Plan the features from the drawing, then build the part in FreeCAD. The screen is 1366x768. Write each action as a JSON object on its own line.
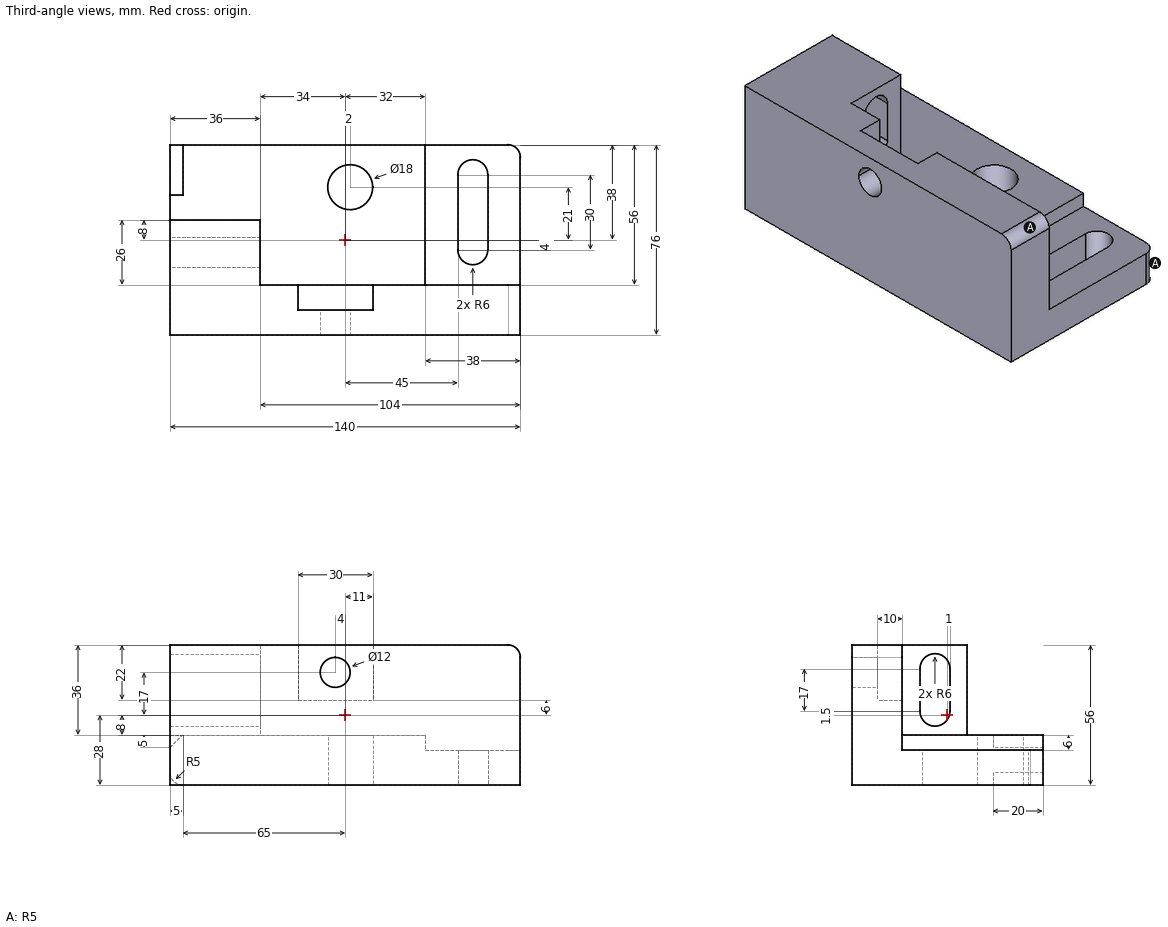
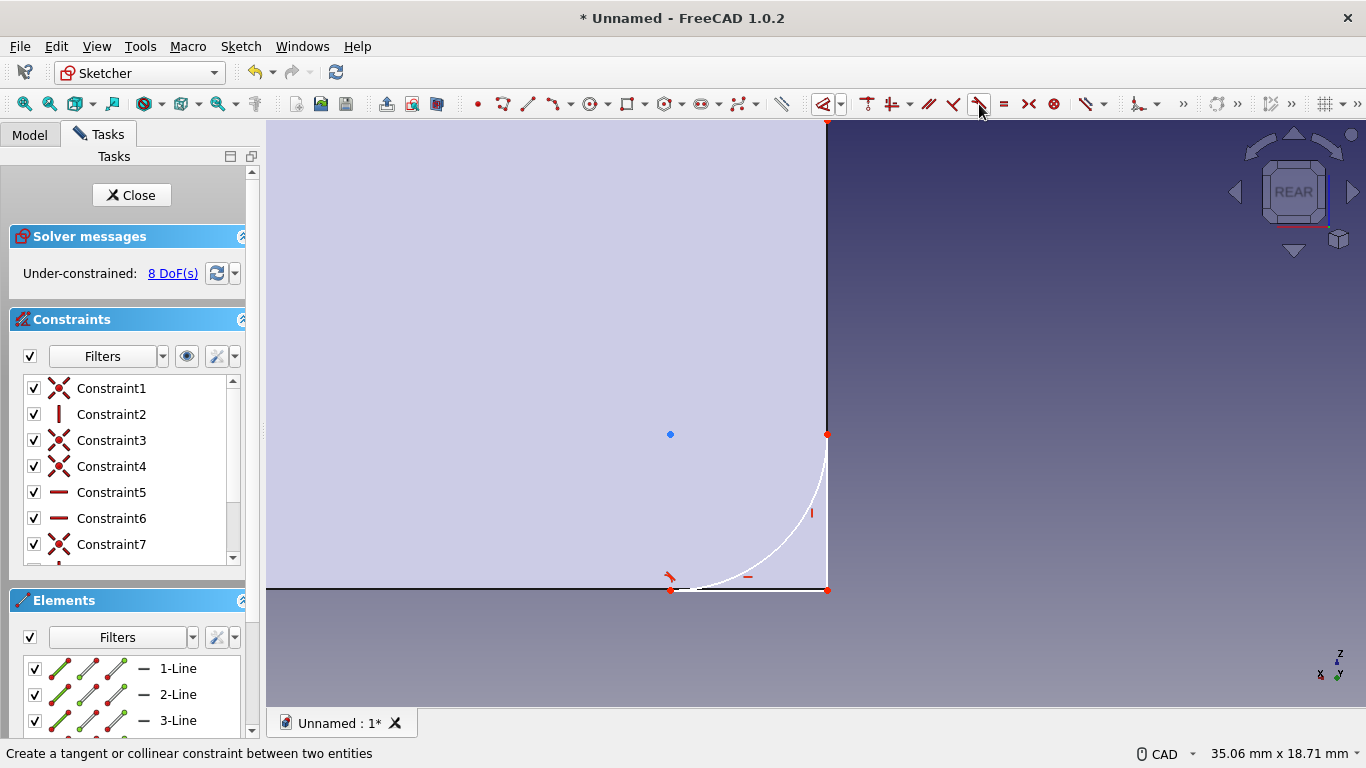
{"action": "left_click", "coordinate": [827, 544]}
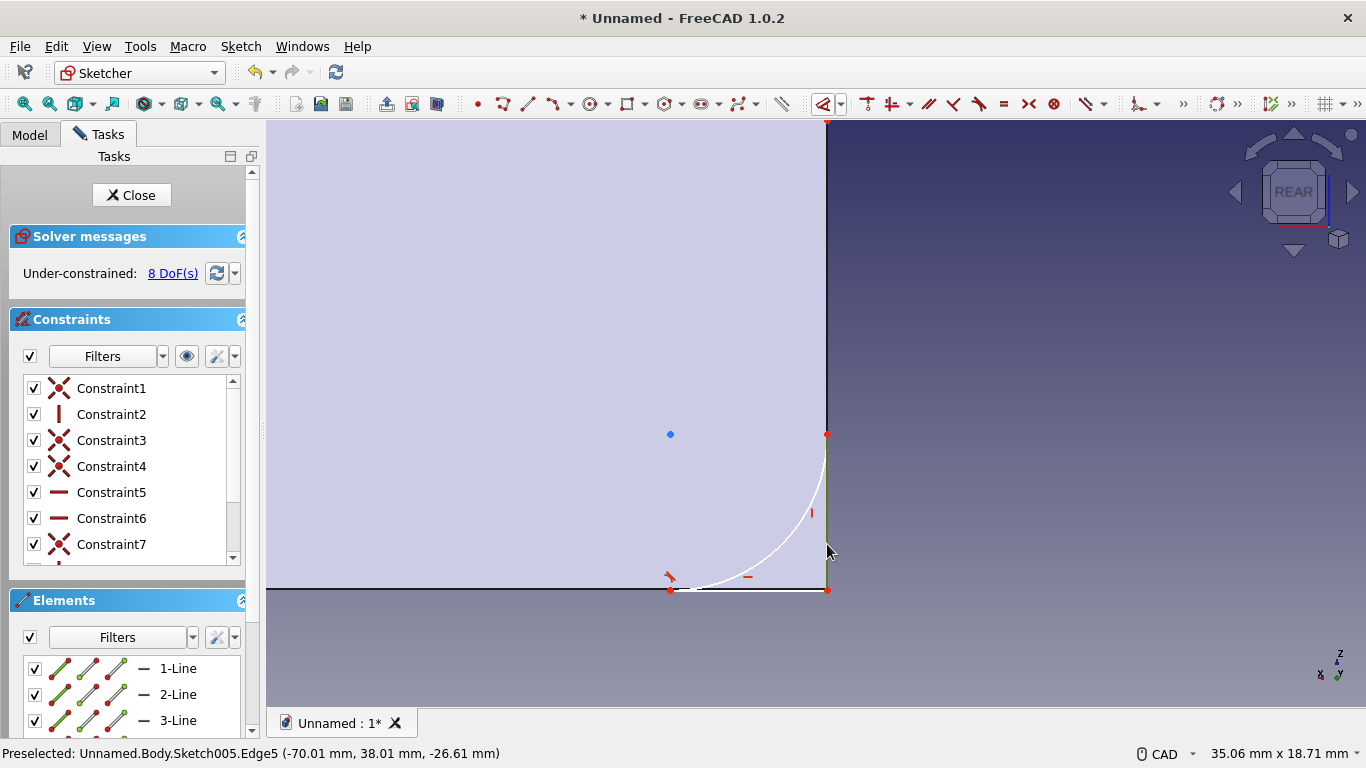
{"action": "left_click", "coordinate": [742, 574]}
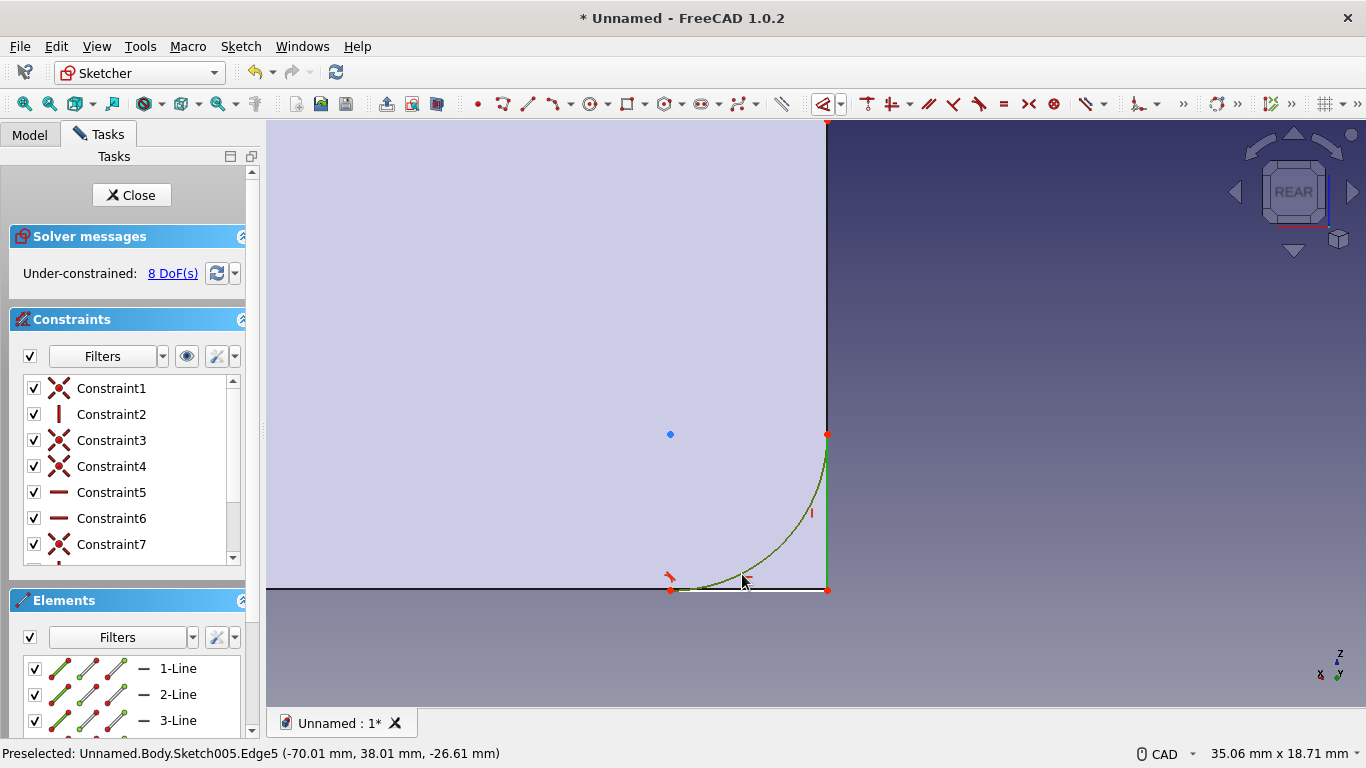
{"action": "left_click", "coordinate": [979, 104]}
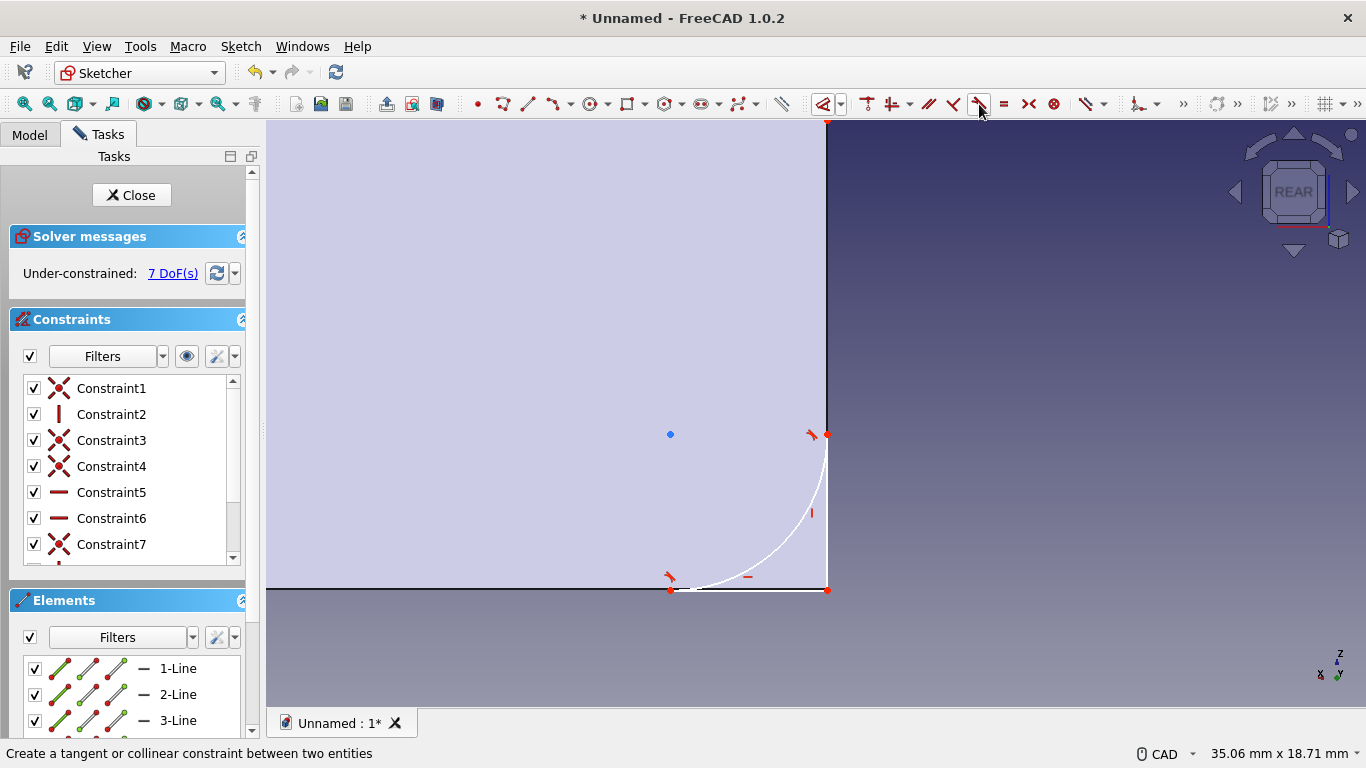
{"action": "left_click", "coordinate": [742, 574]}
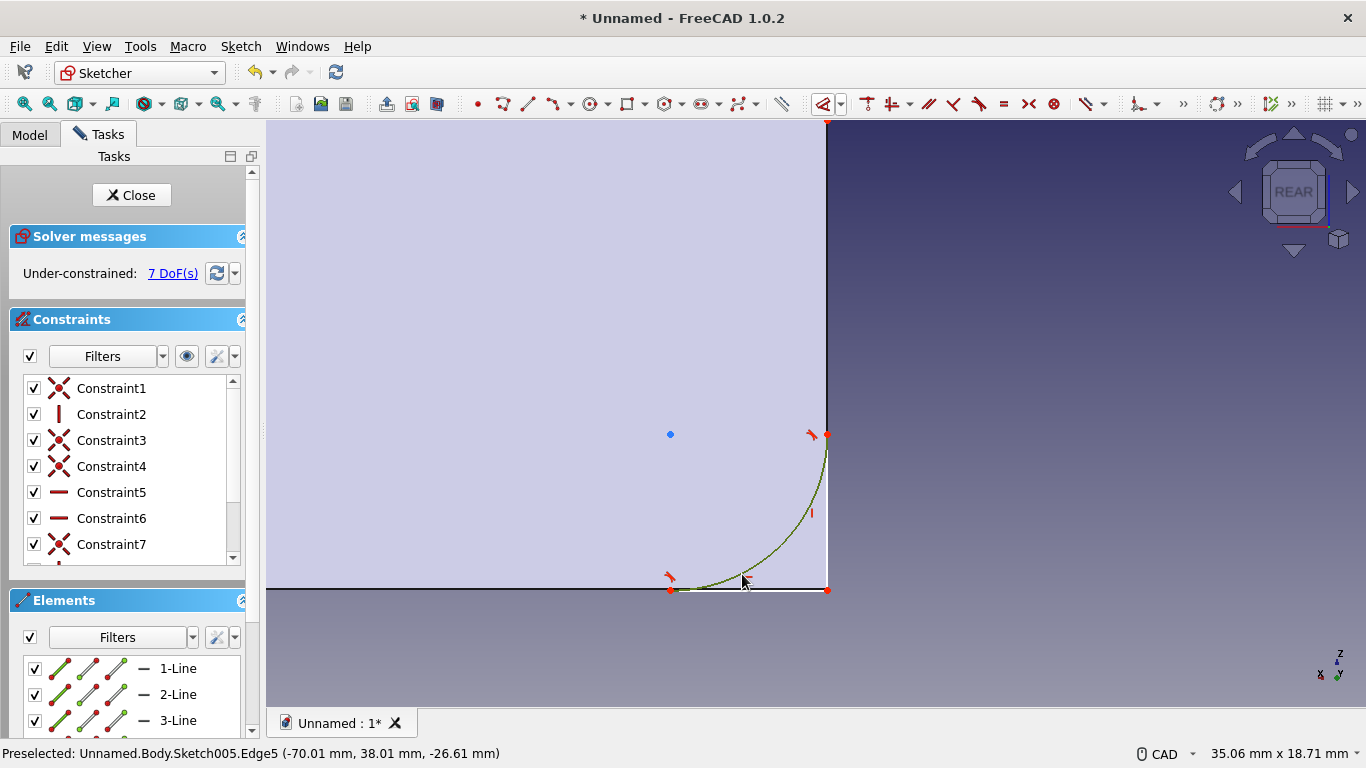
{"action": "key", "text": "k r"}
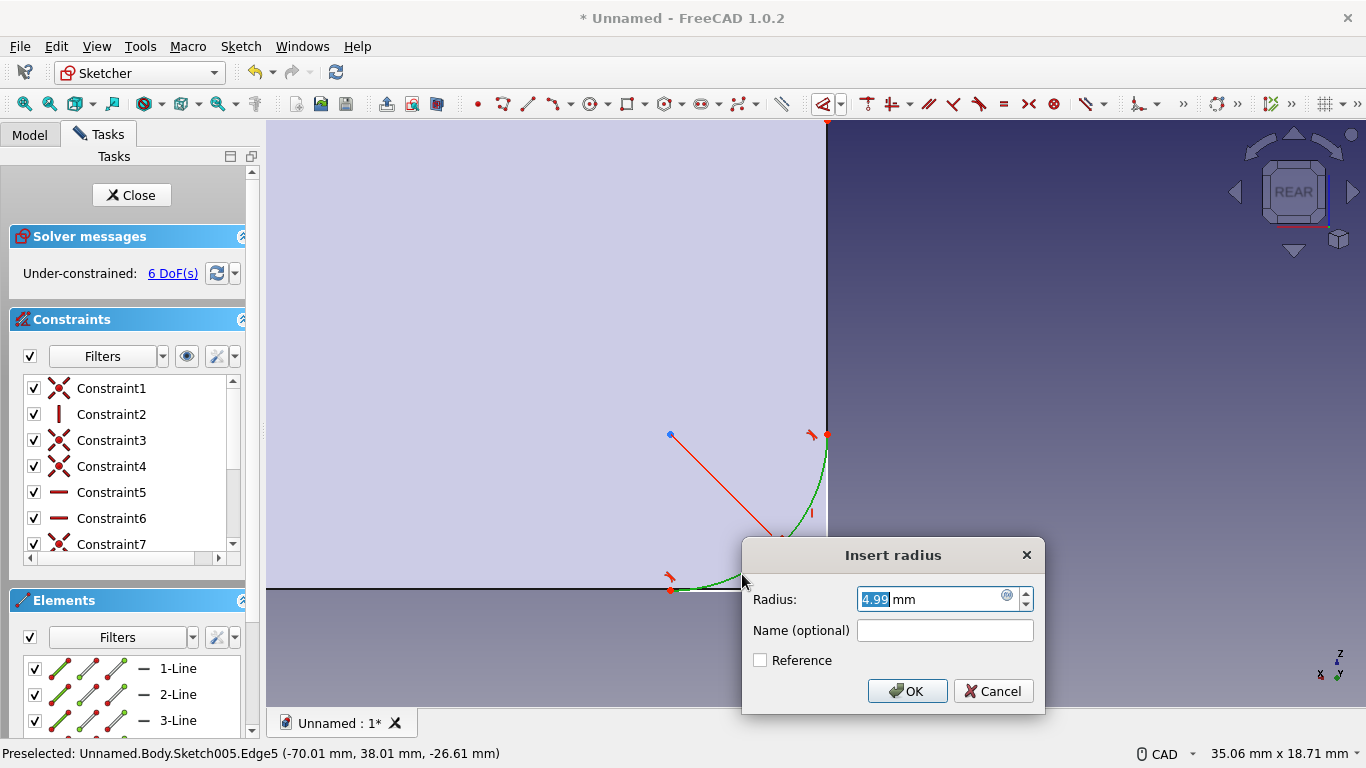
{"action": "type", "text": "5"}
{"action": "key", "text": "Return"}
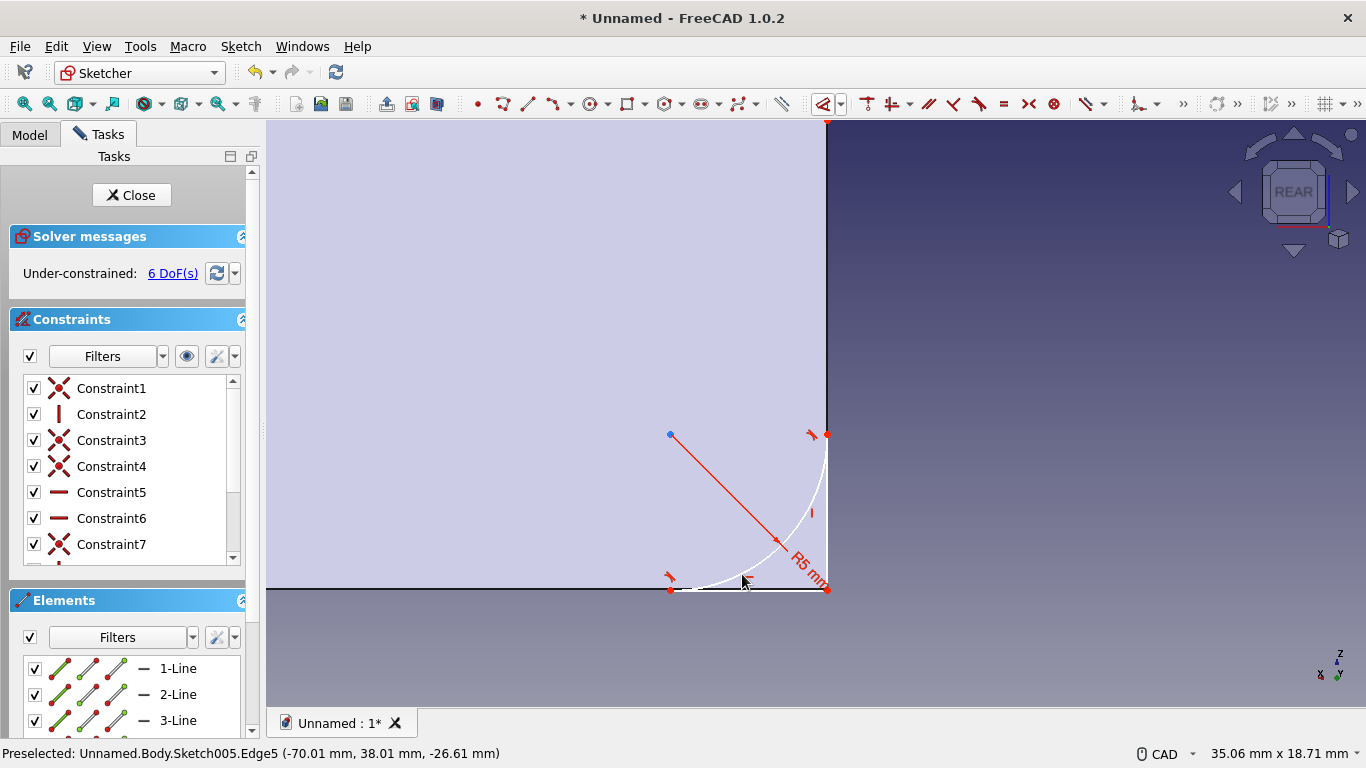
{"action": "scroll", "coordinate": [746, 582], "scroll_direction": "down", "scroll_amount": 3}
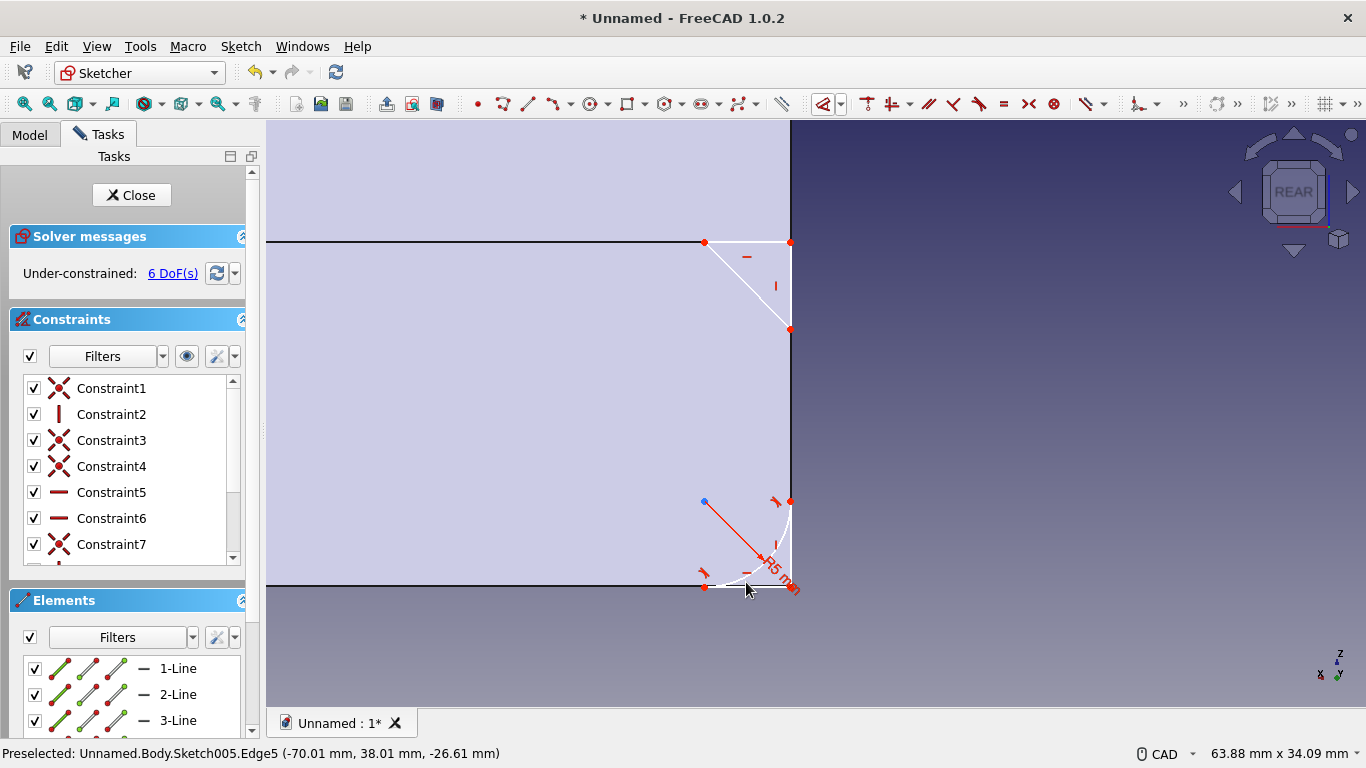
{"action": "left_click", "coordinate": [791, 303]}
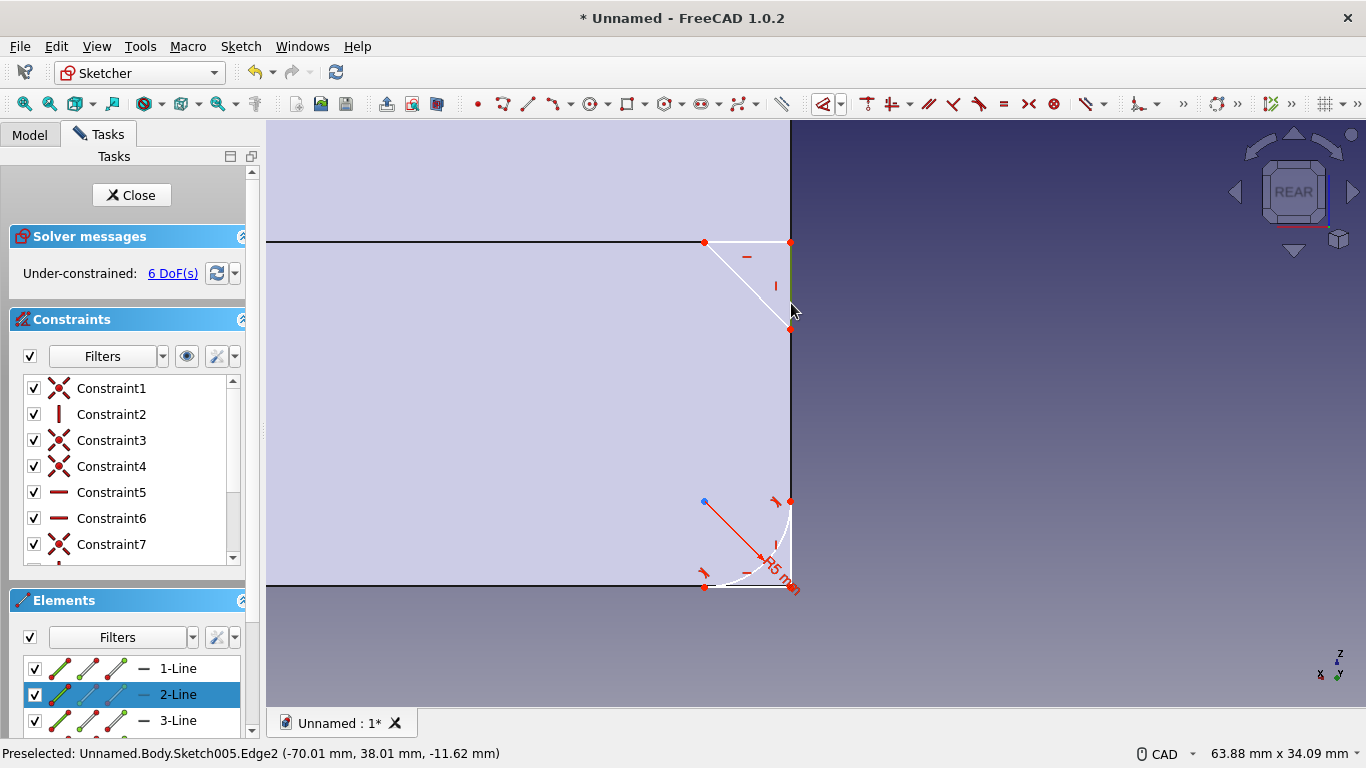
{"action": "key", "text": "i"}